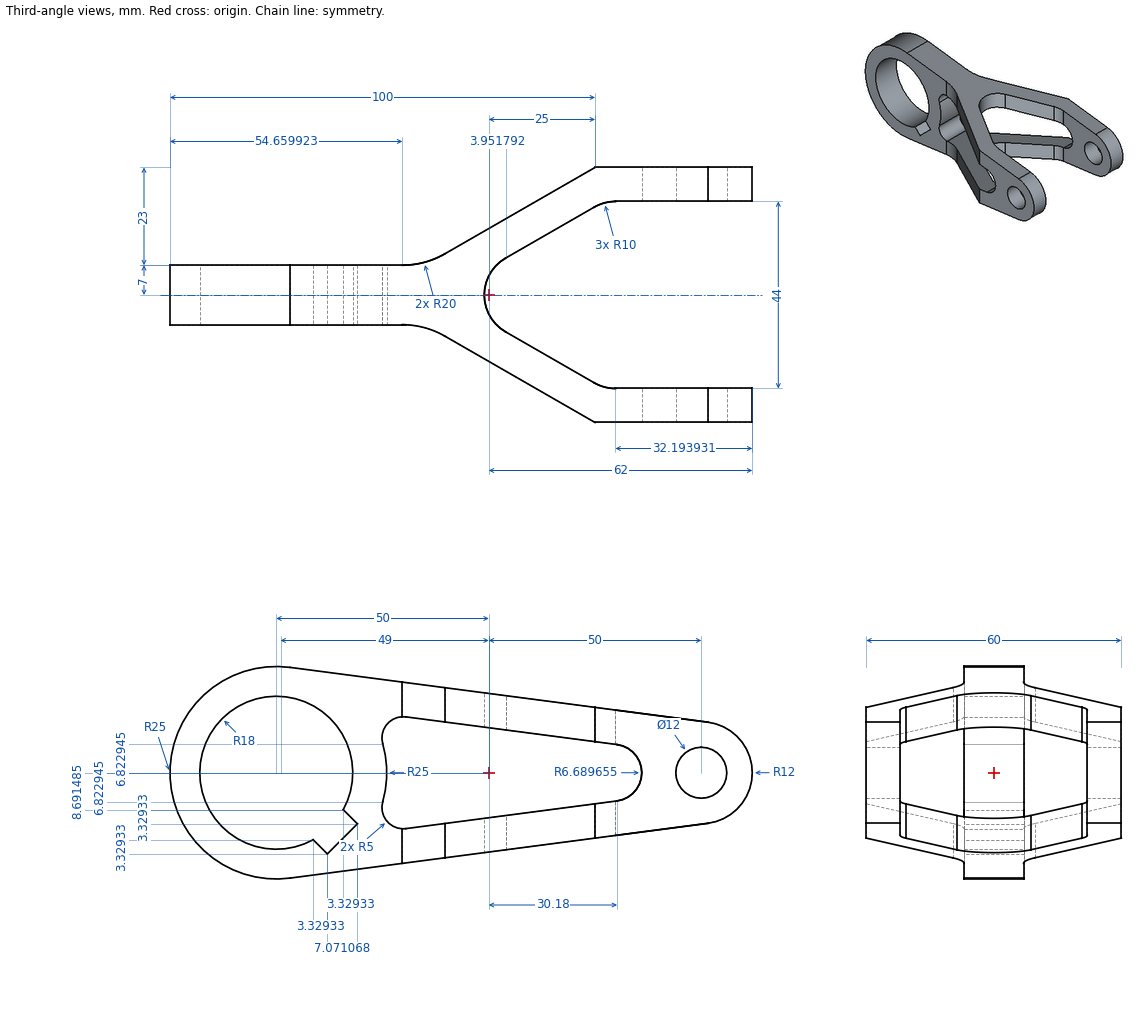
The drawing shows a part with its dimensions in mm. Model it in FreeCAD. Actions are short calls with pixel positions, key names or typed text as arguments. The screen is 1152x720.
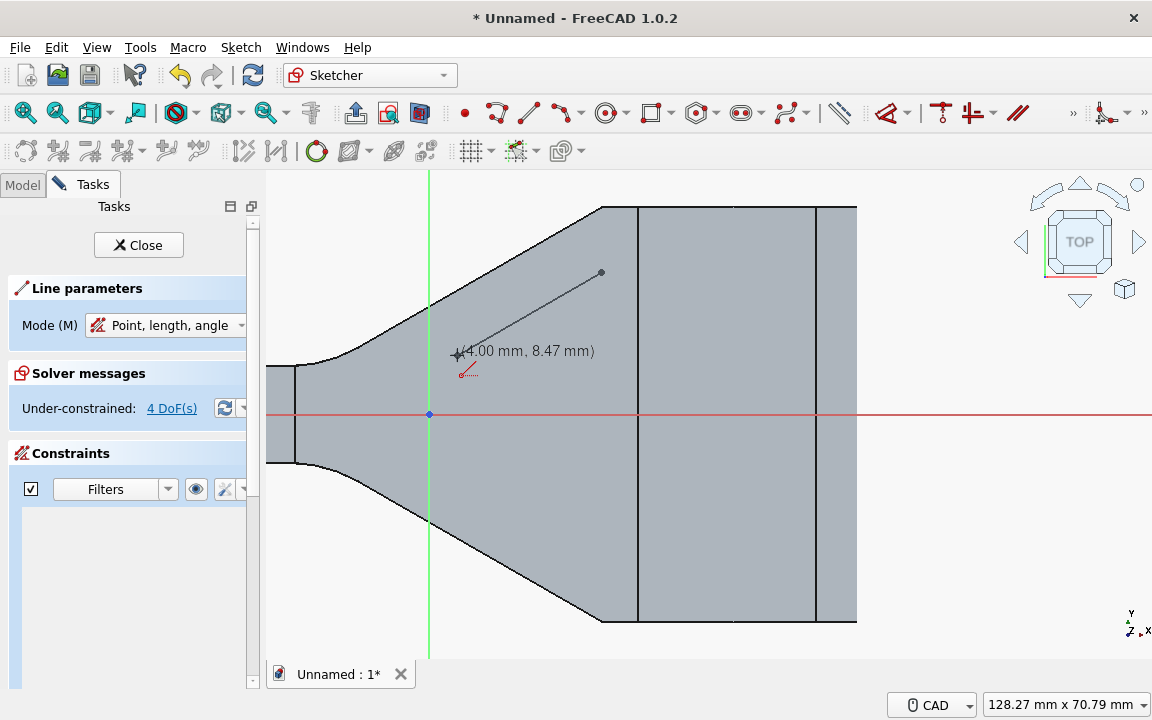
click(457, 474)
click(601, 557)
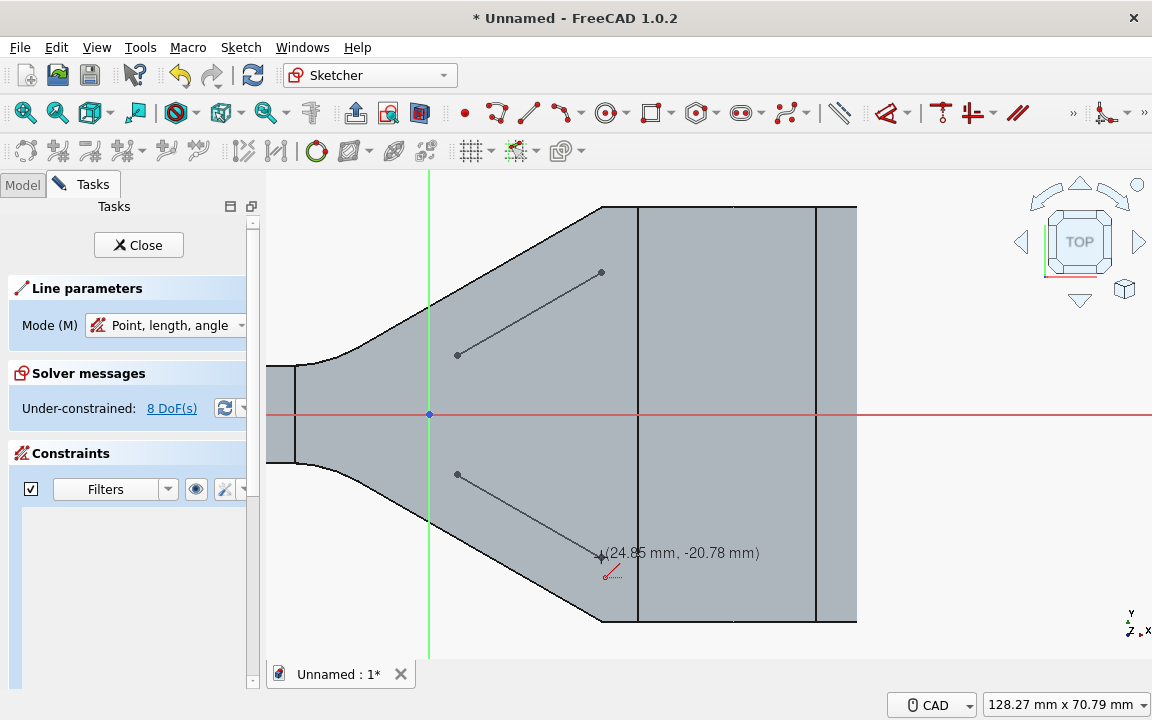
click(498, 114)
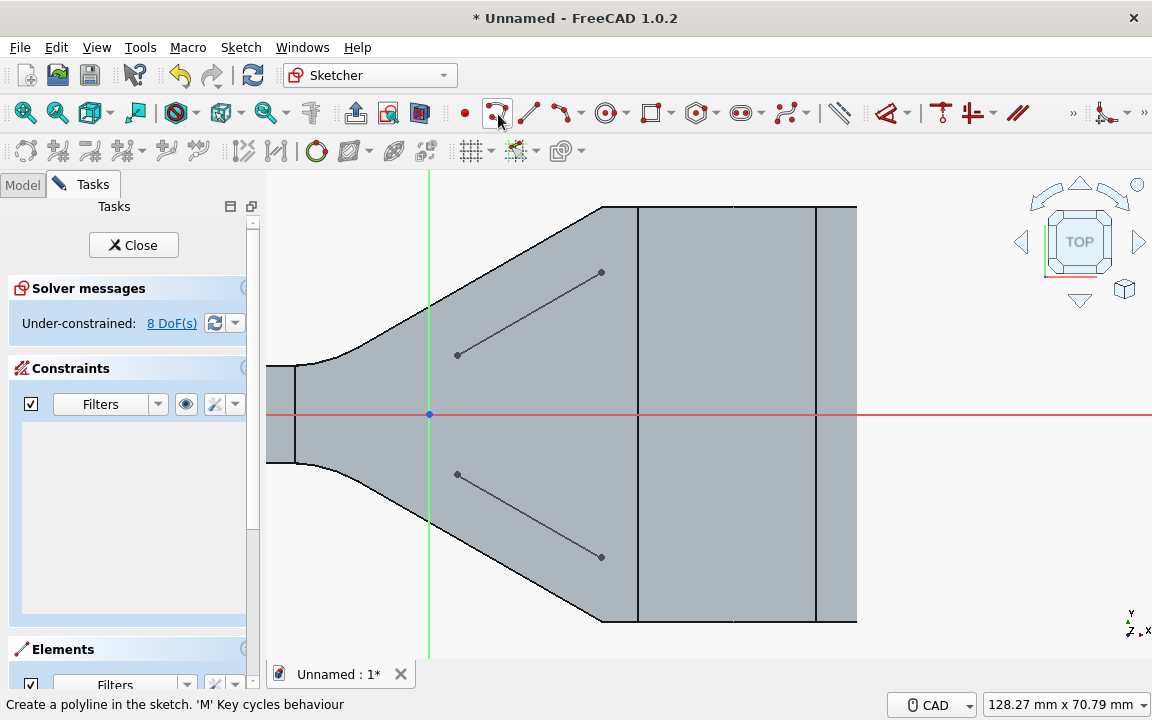
click(635, 566)
click(858, 566)
click(858, 263)
click(635, 263)
right_click(635, 263)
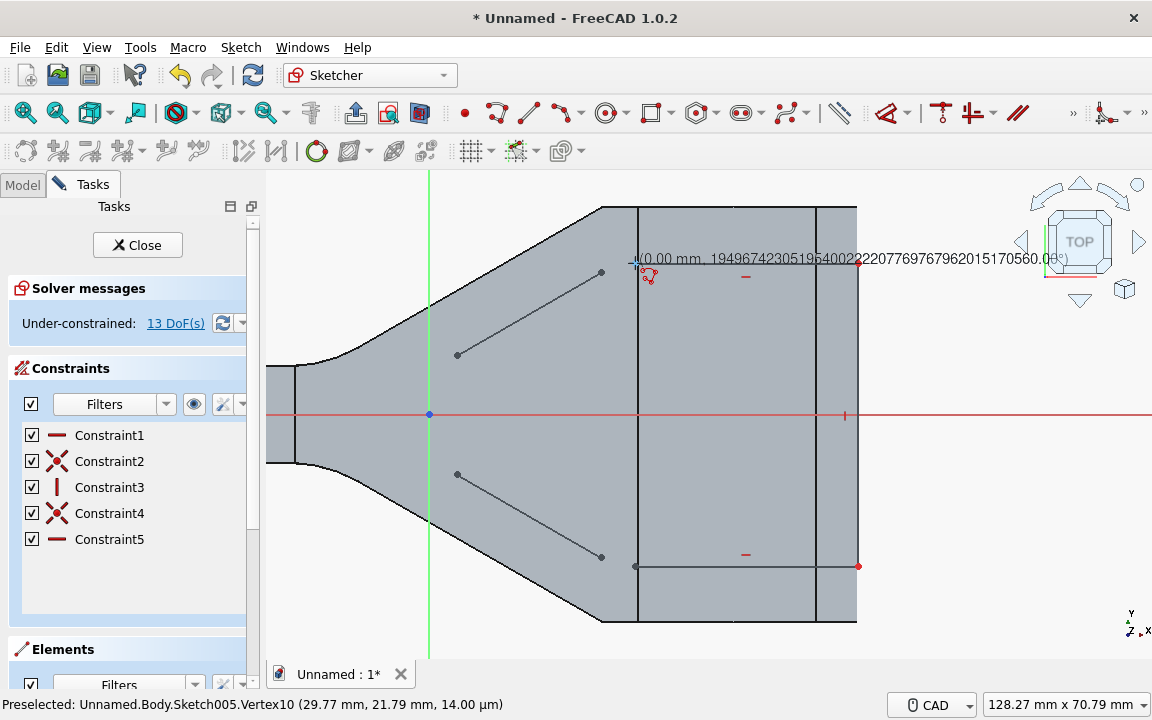
click(562, 114)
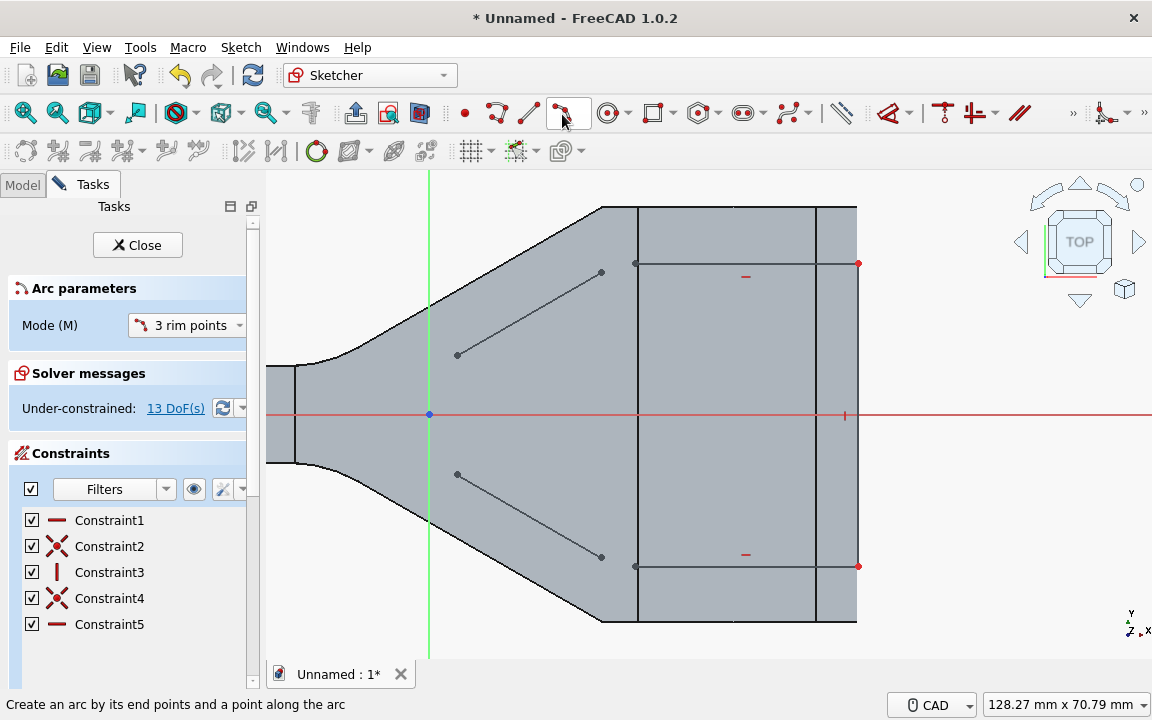
click(457, 356)
click(457, 475)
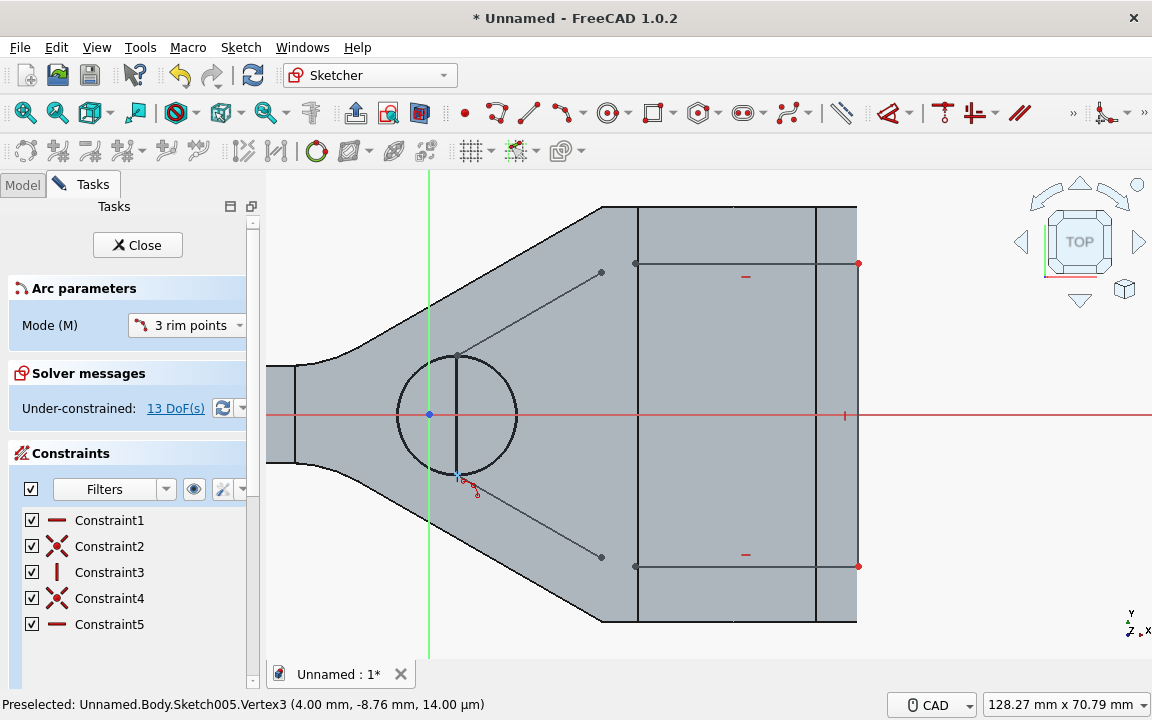
scroll(424, 429, up, 6)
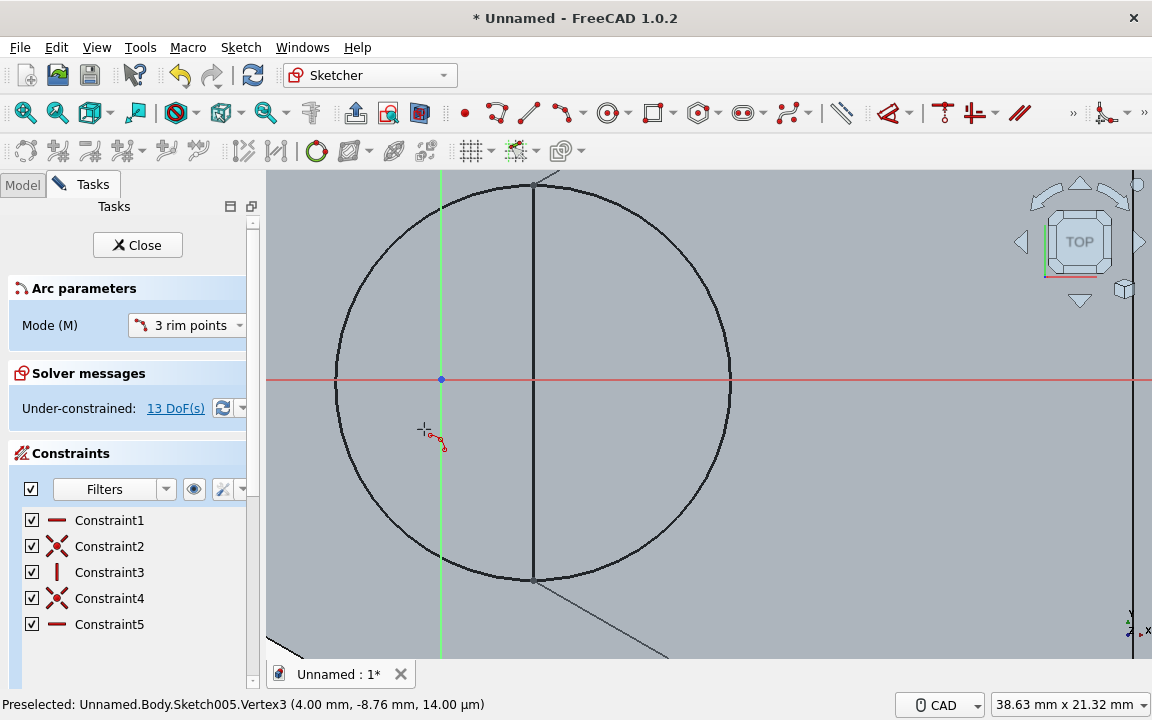
click(422, 427)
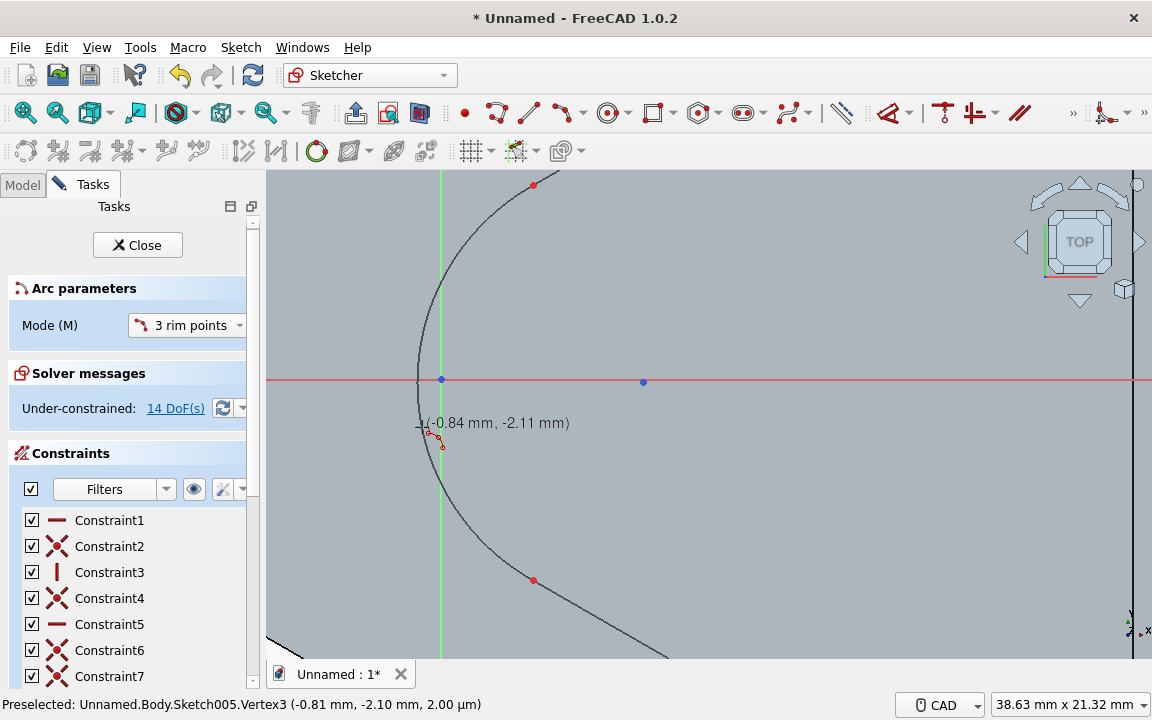
scroll(425, 430, down, 6)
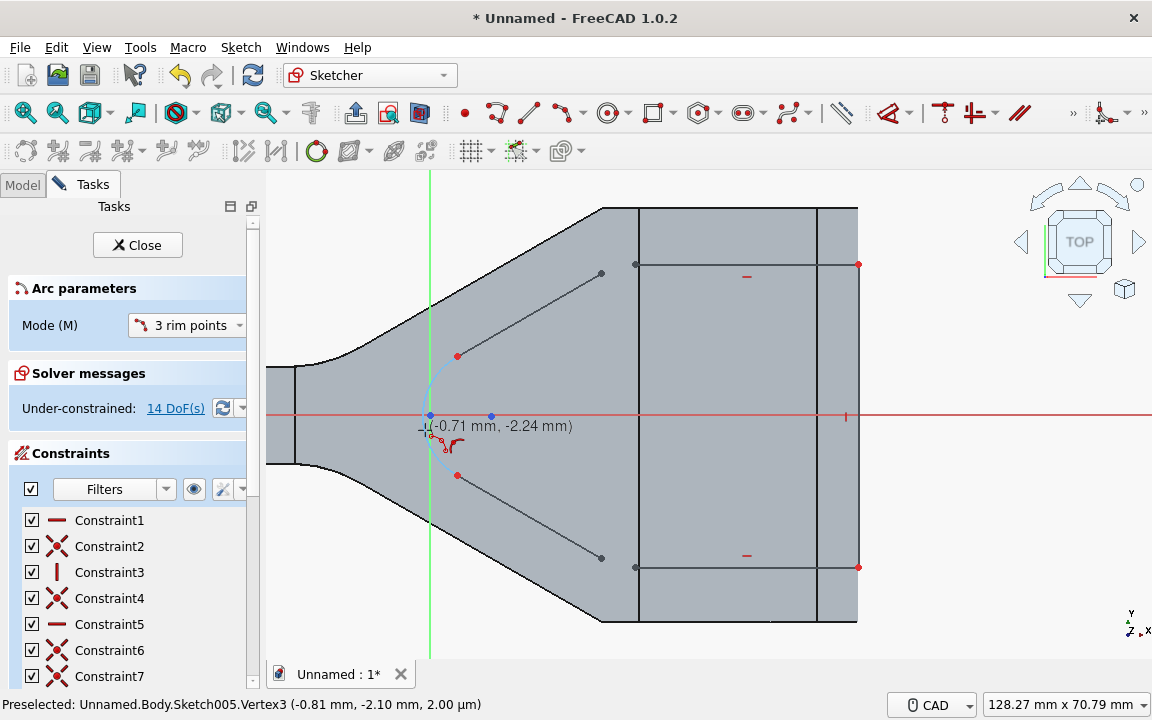
click(602, 559)
click(636, 568)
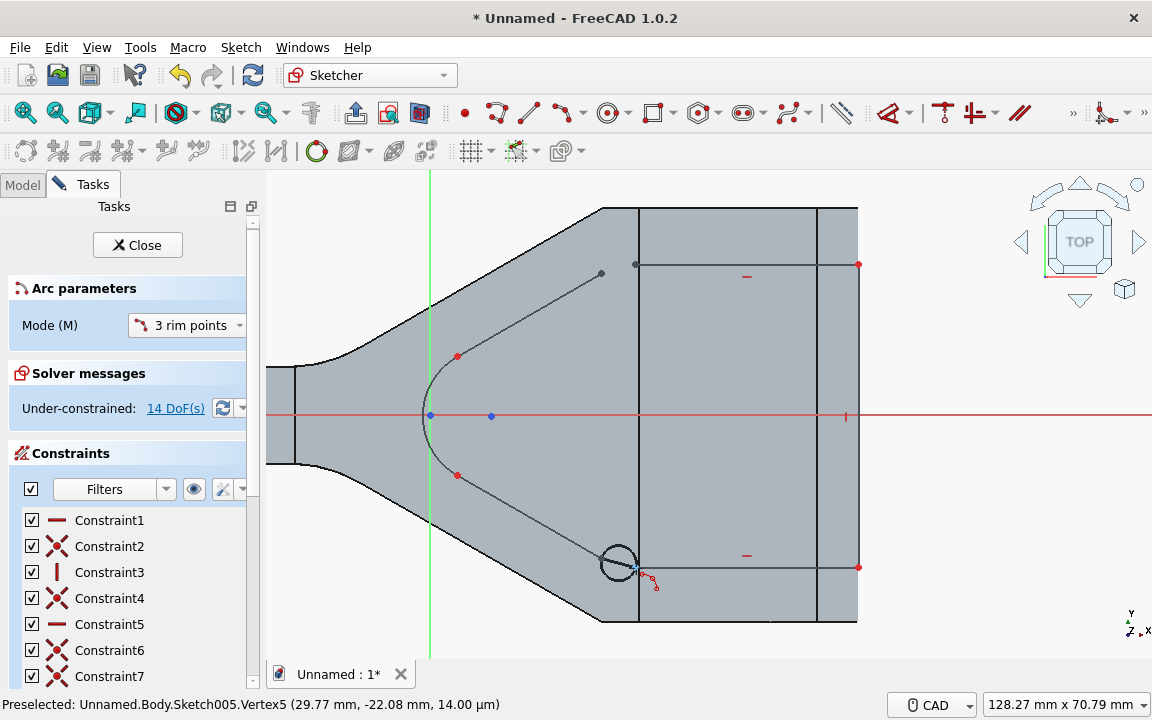
scroll(618, 565, up, 10)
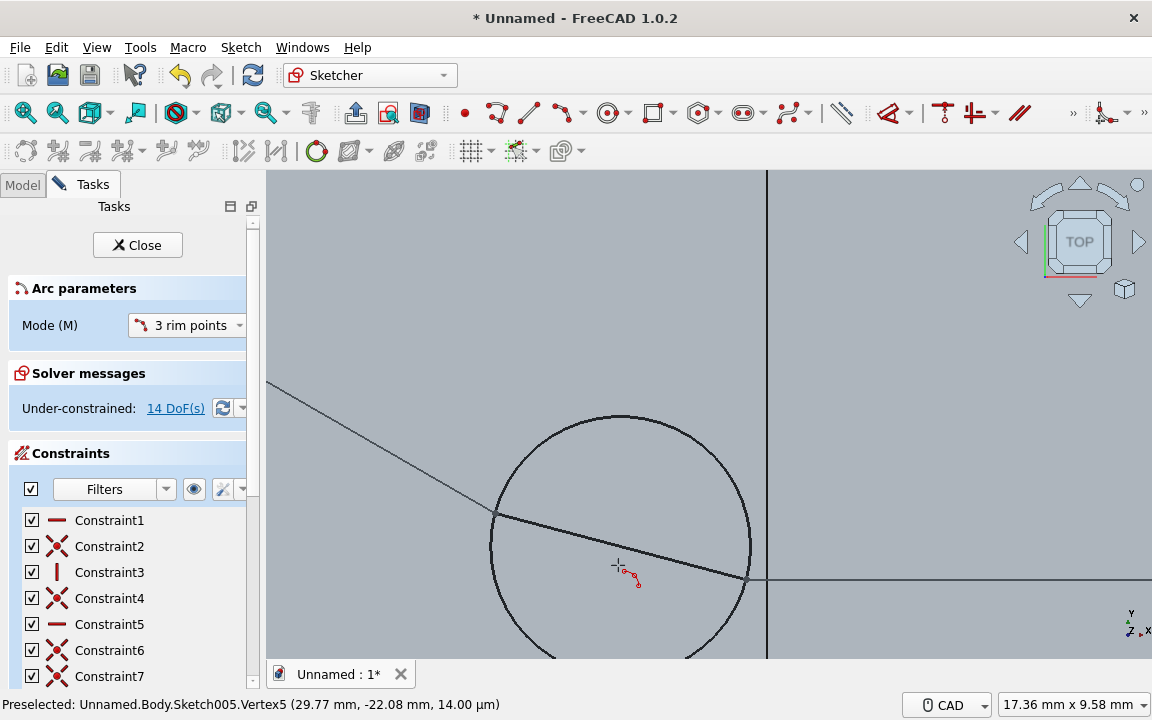
click(616, 559)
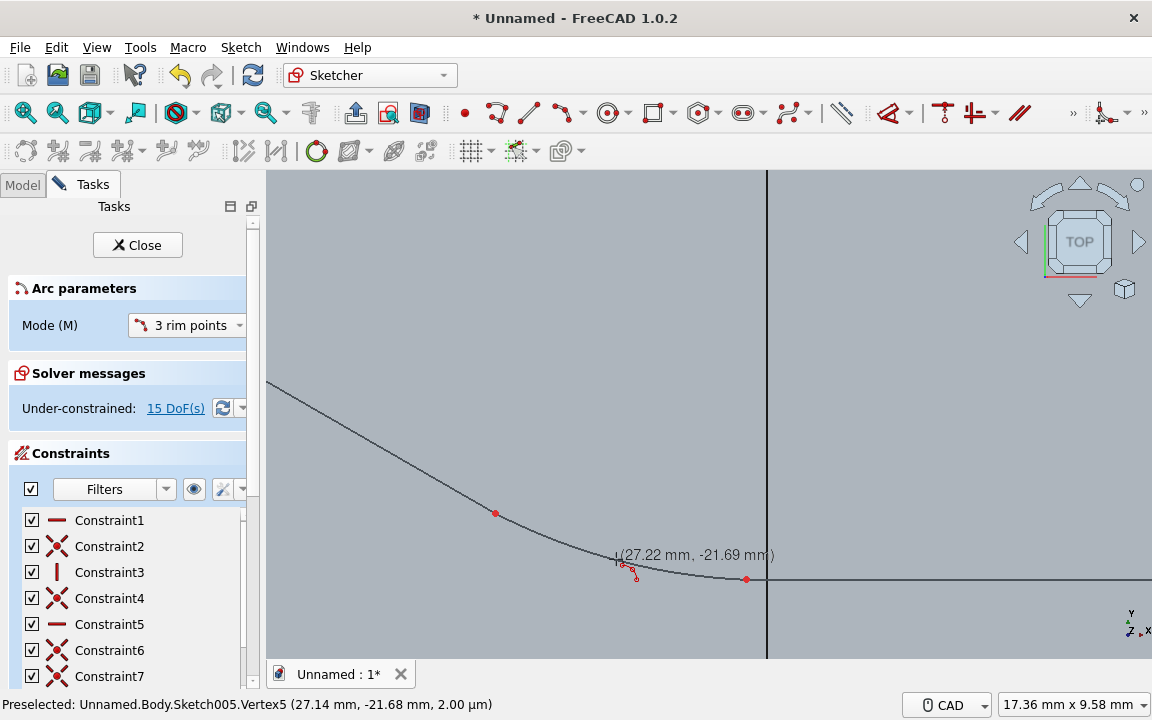
scroll(618, 565, down, 10)